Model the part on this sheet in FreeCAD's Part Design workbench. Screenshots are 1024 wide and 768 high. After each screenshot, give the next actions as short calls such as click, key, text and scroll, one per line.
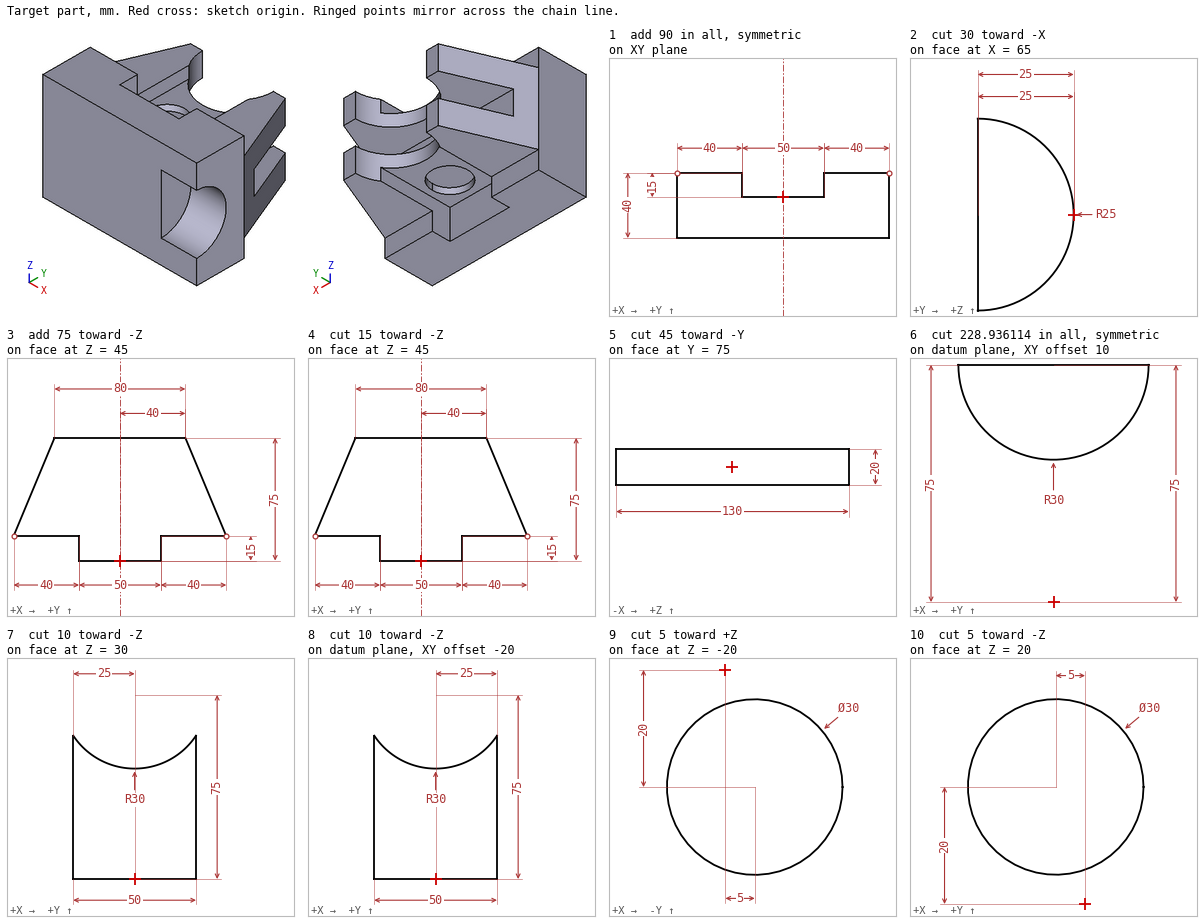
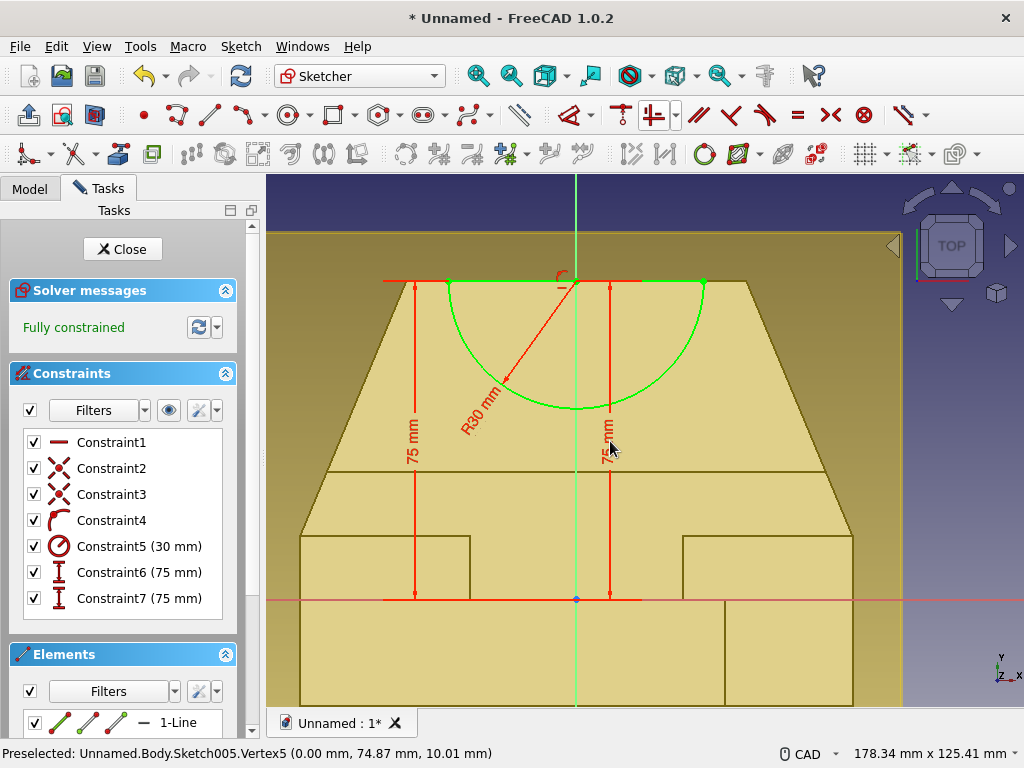
click(123, 249)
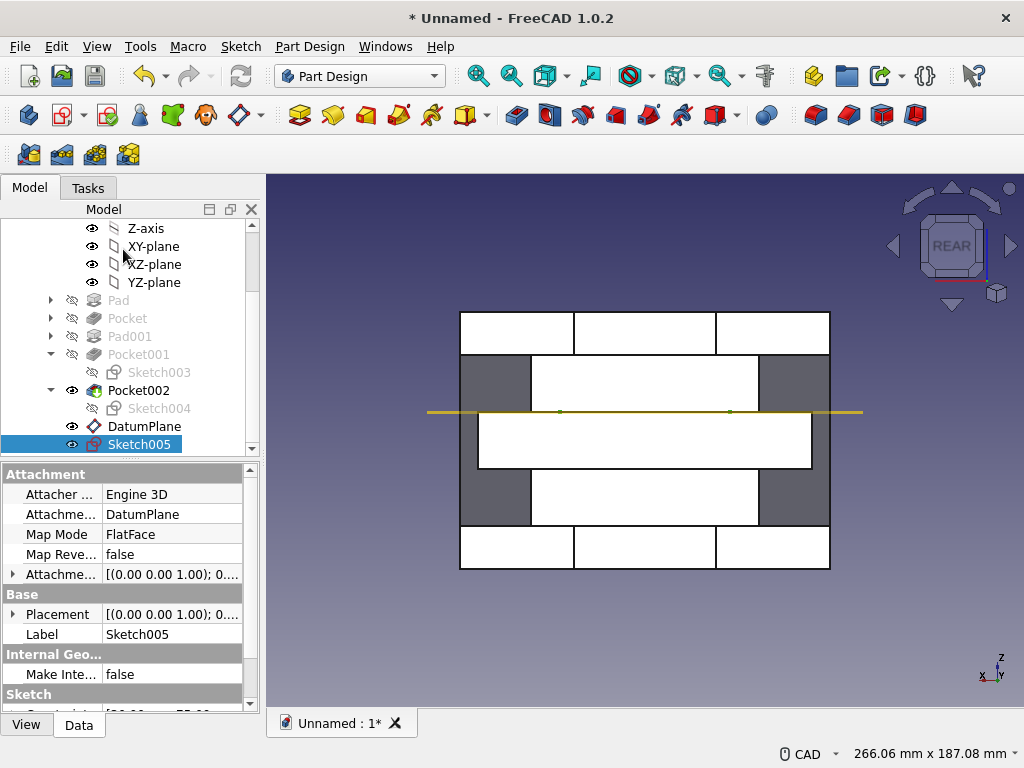
click(517, 116)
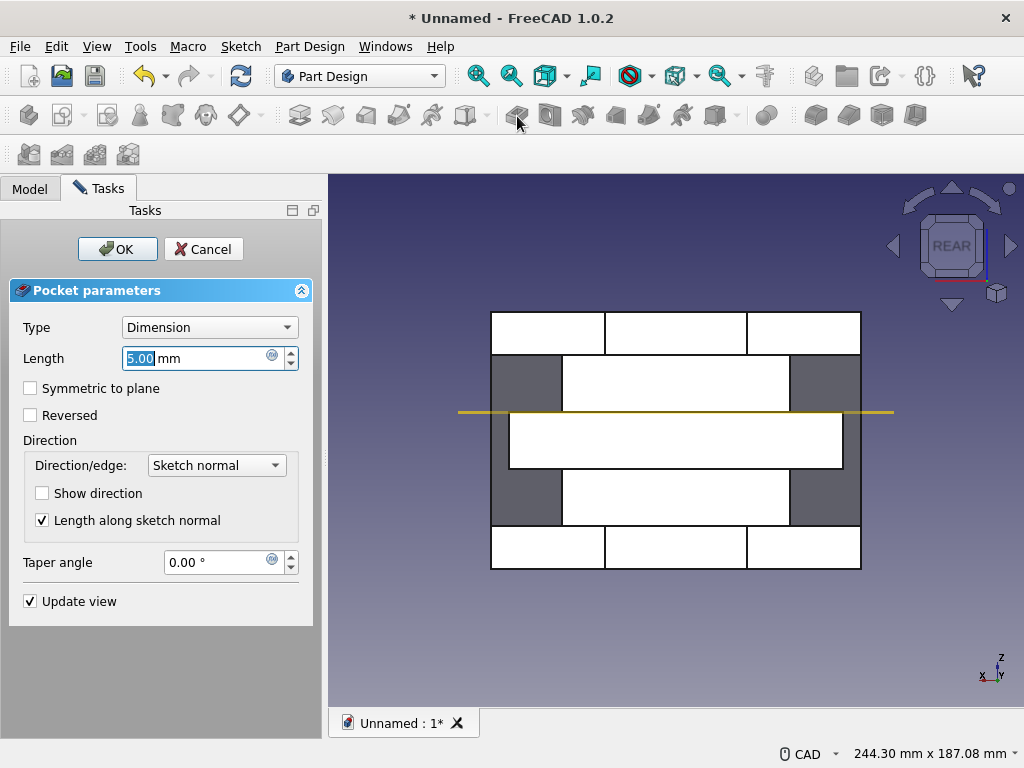
text(228.936114)
key(Tab)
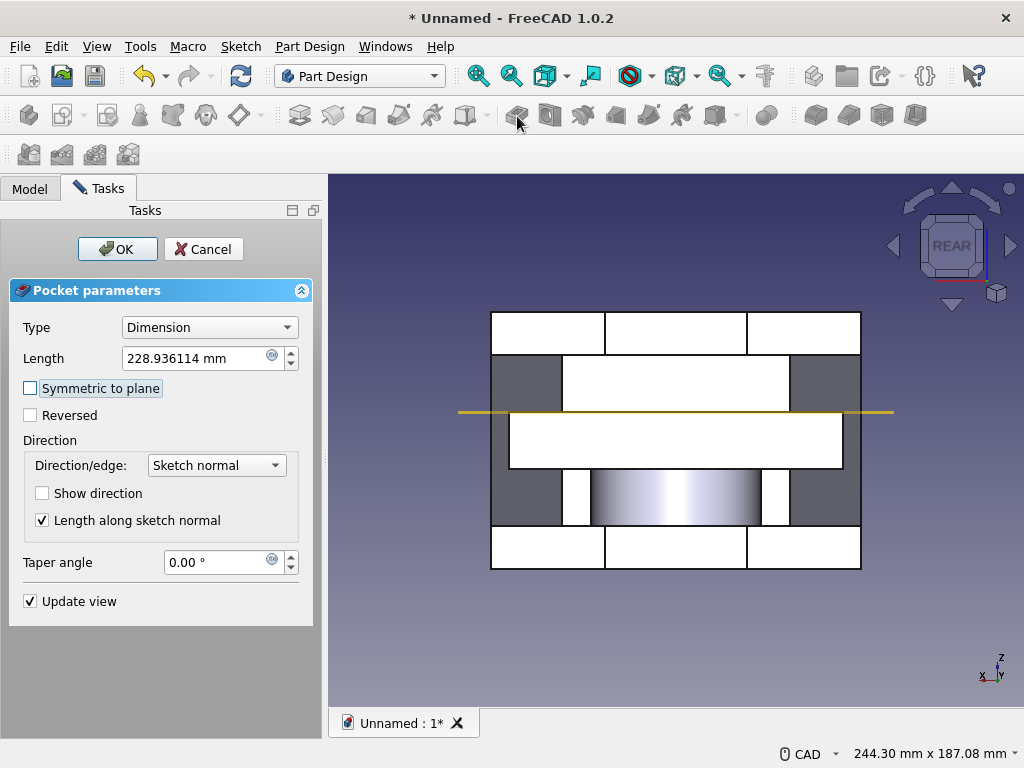
click(31, 388)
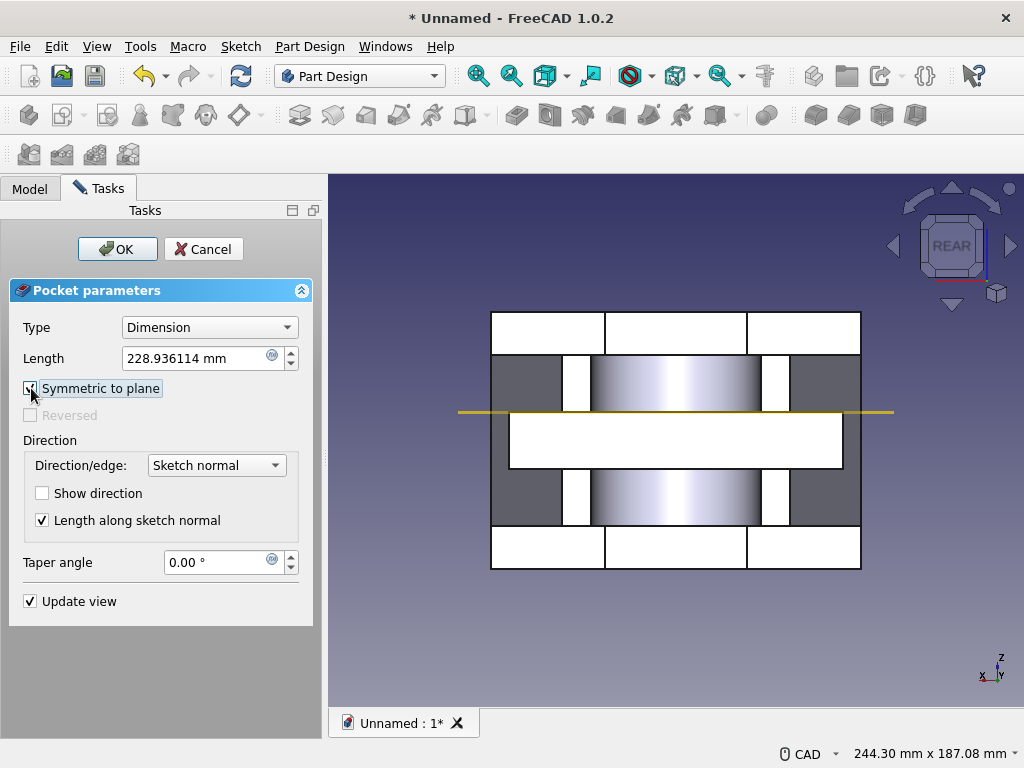
click(118, 249)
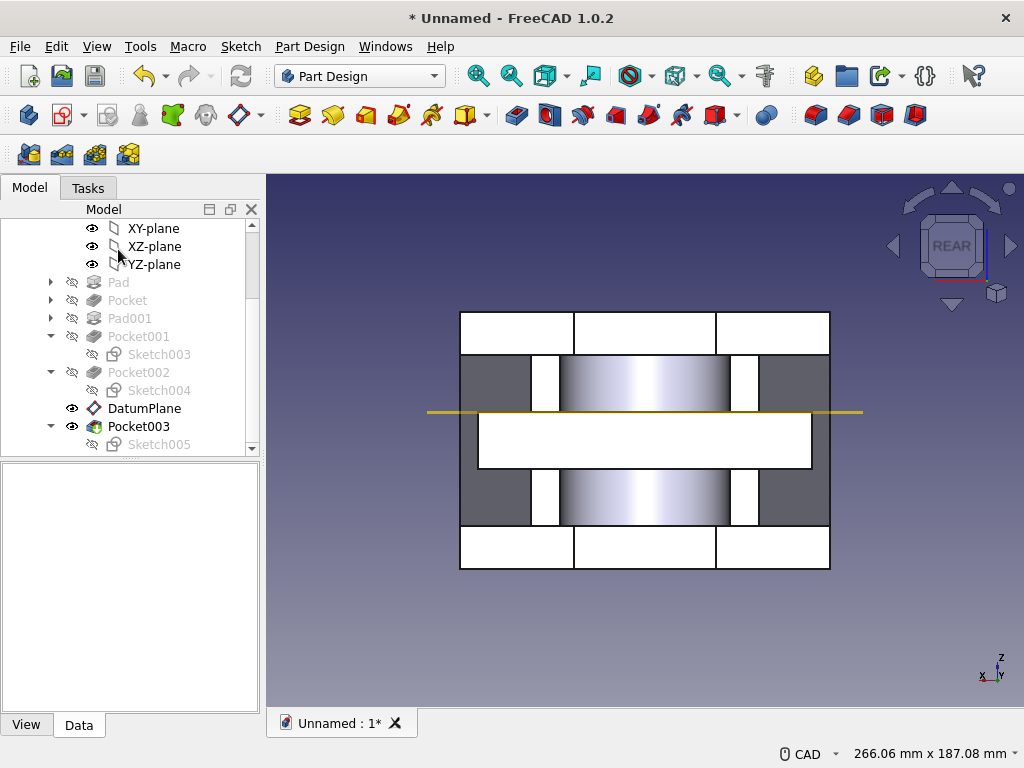
click(117, 408)
key(space)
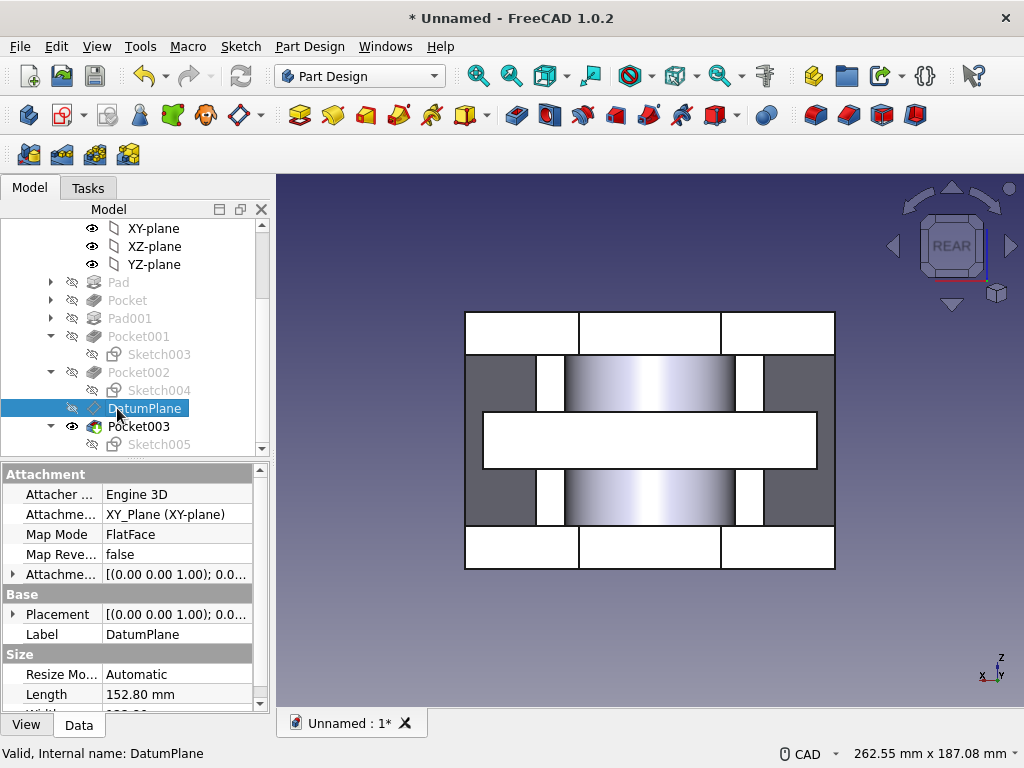
key(0)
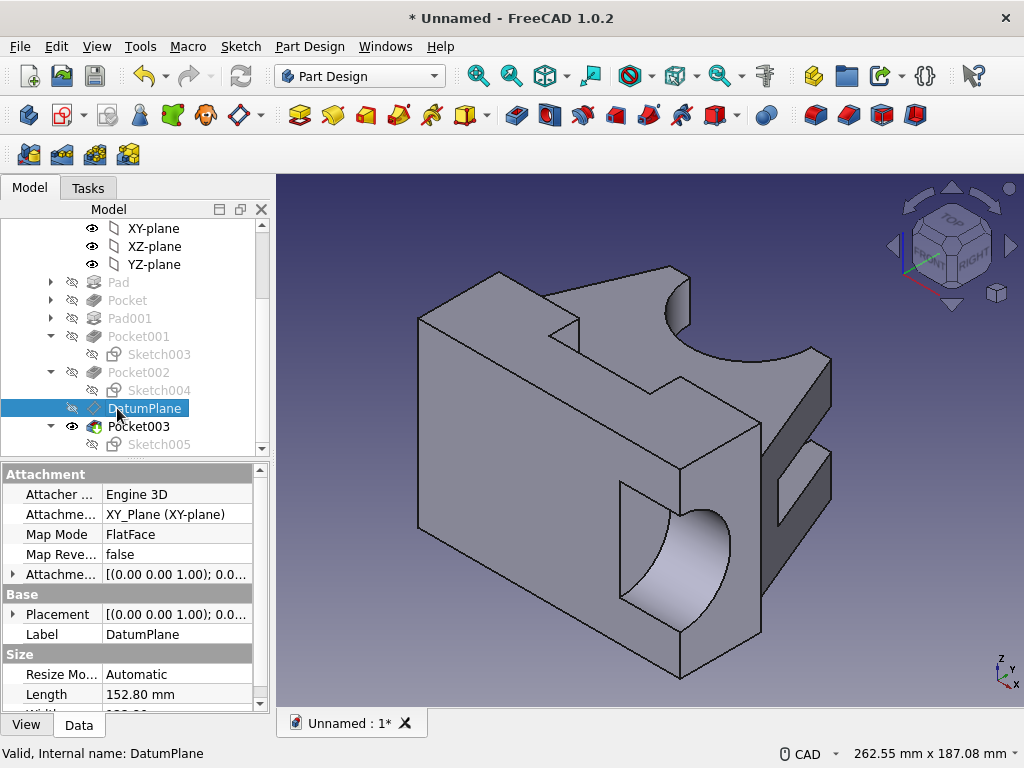
click(654, 368)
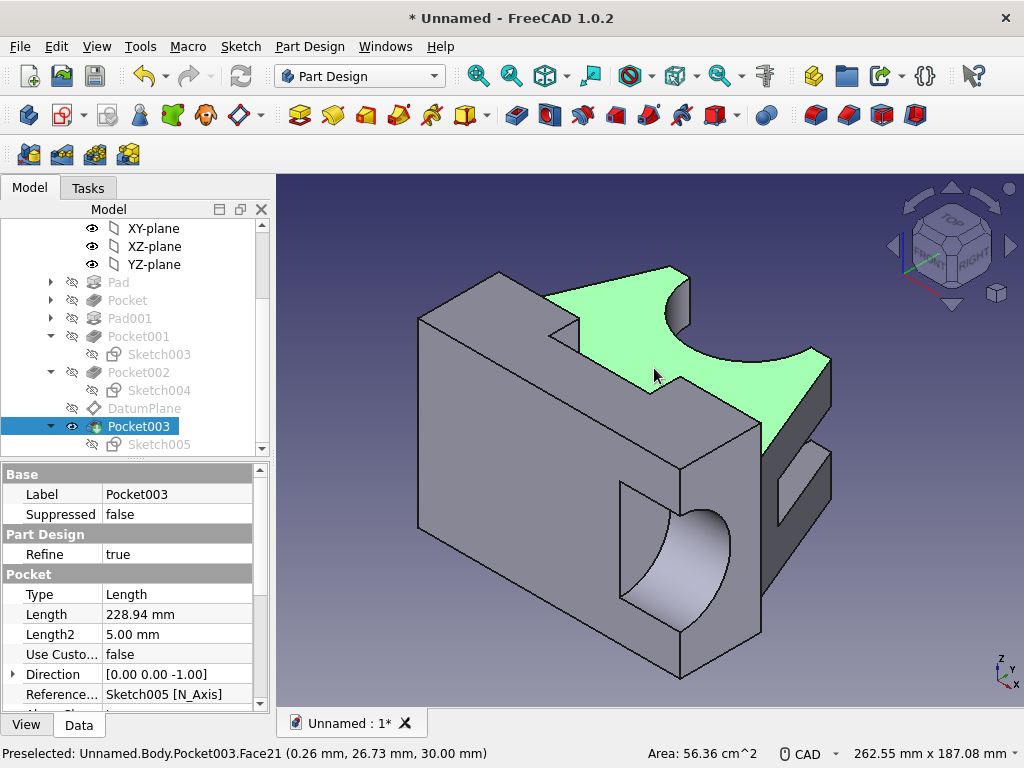
click(62, 116)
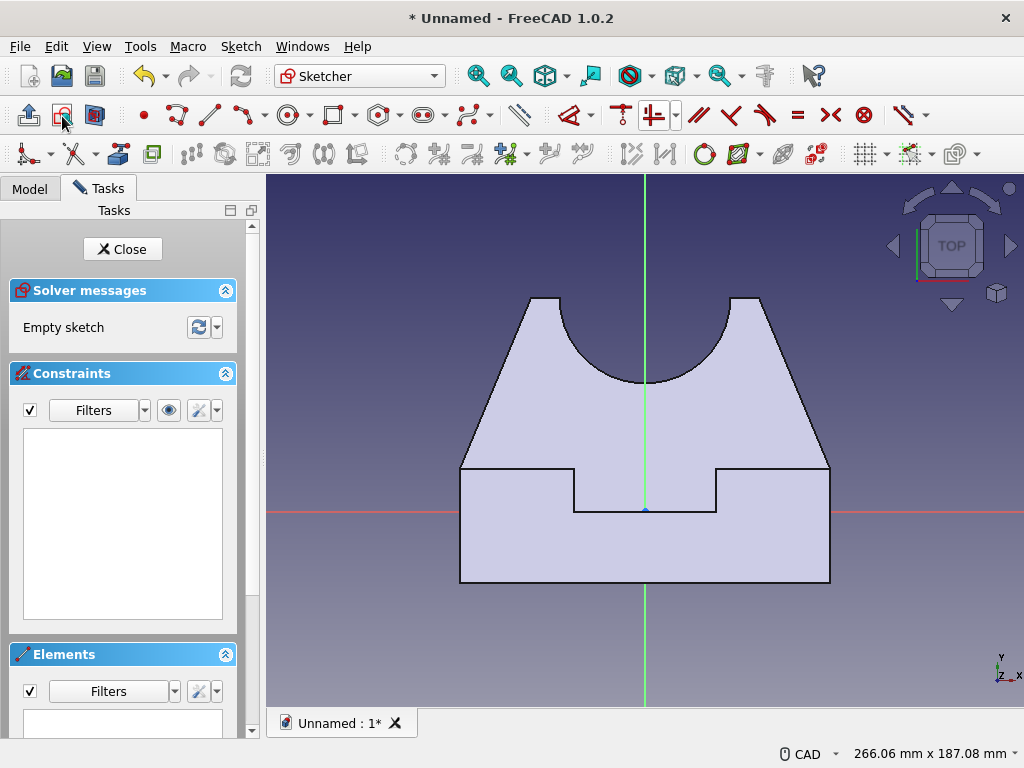
key(q)
key(s)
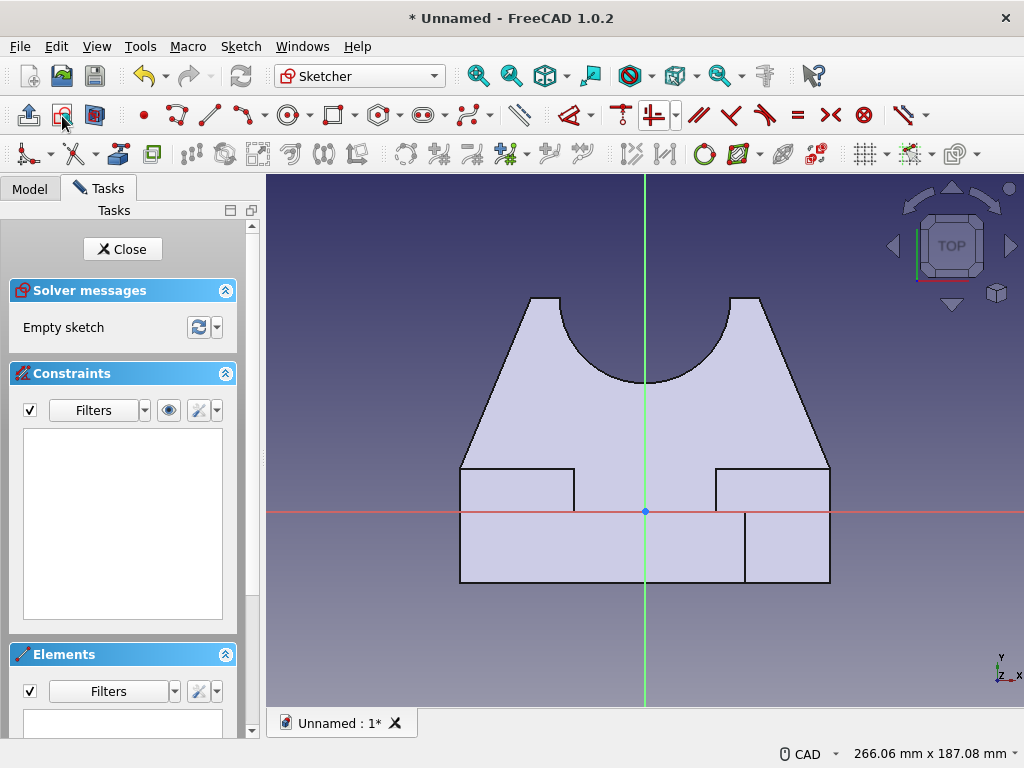
scroll(701, 419, up, 4)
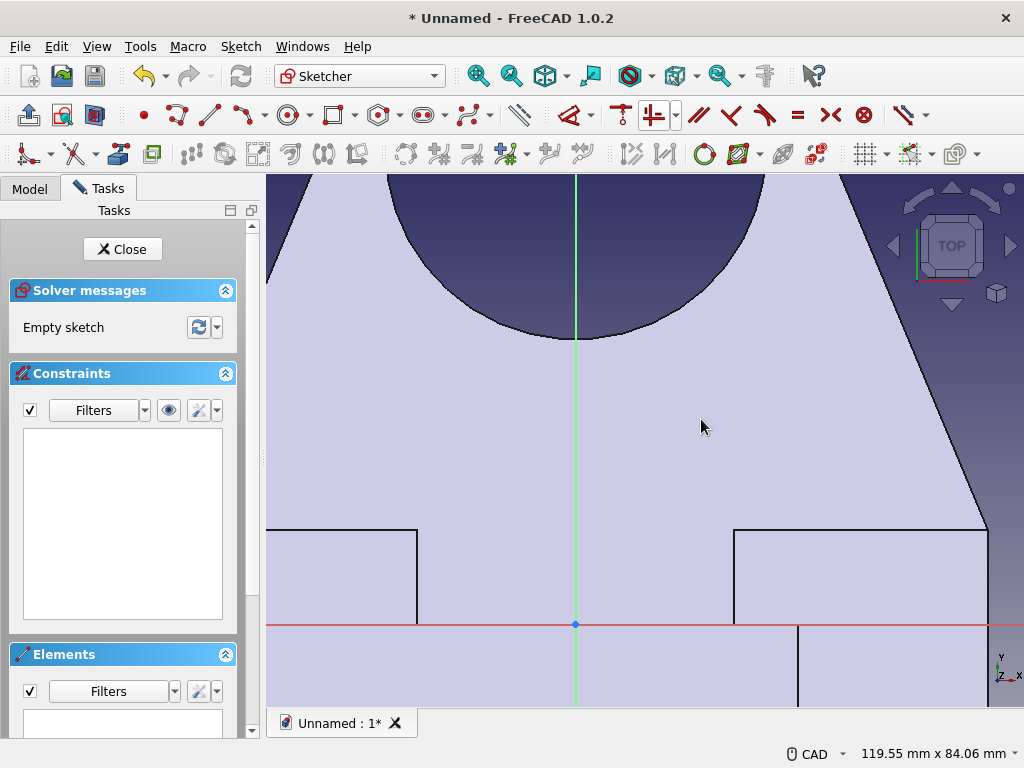
click(177, 116)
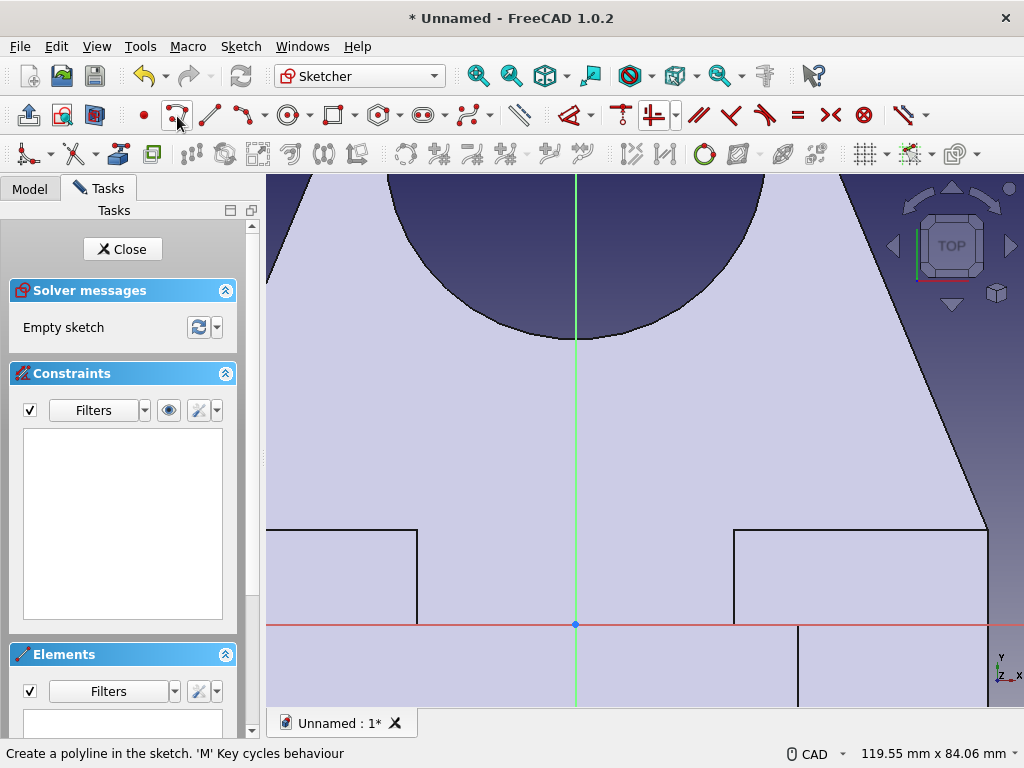
click(417, 254)
click(417, 625)
click(734, 616)
click(734, 254)
right_click(734, 254)